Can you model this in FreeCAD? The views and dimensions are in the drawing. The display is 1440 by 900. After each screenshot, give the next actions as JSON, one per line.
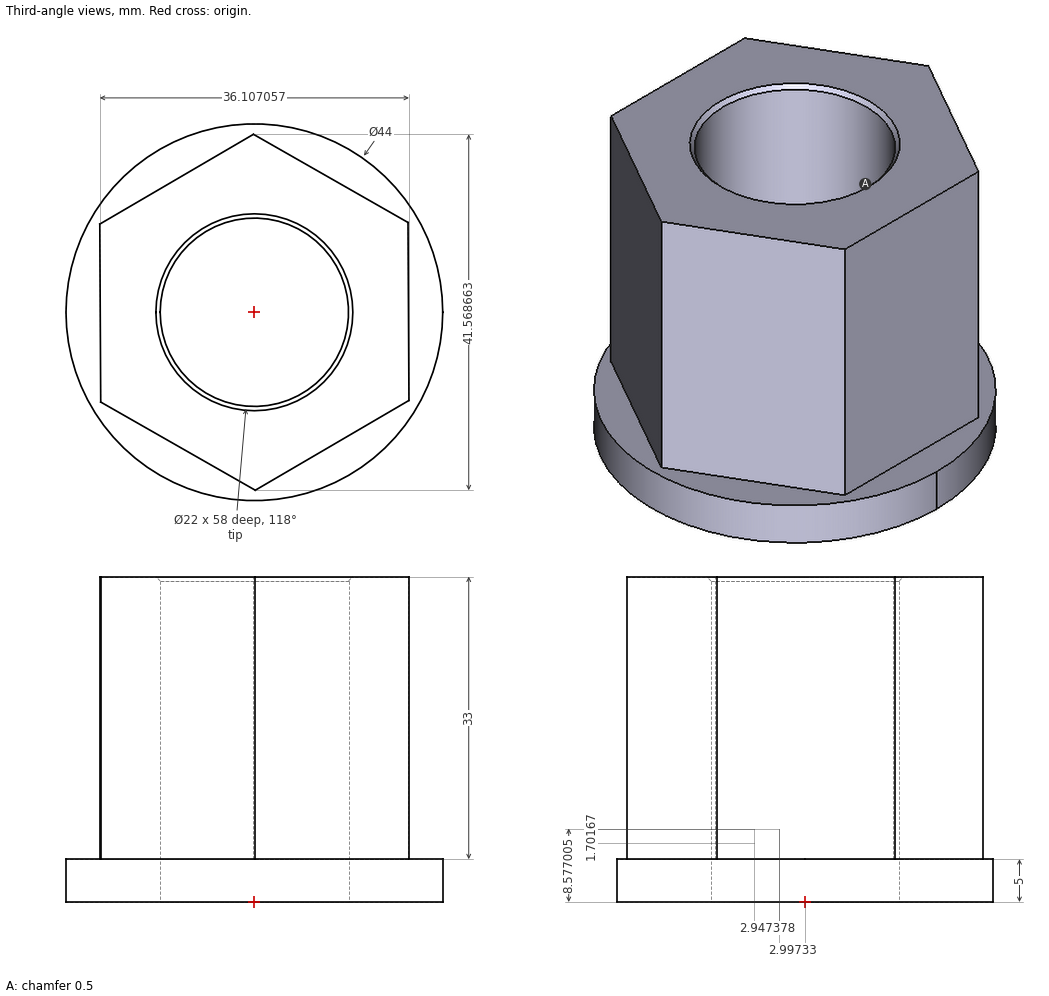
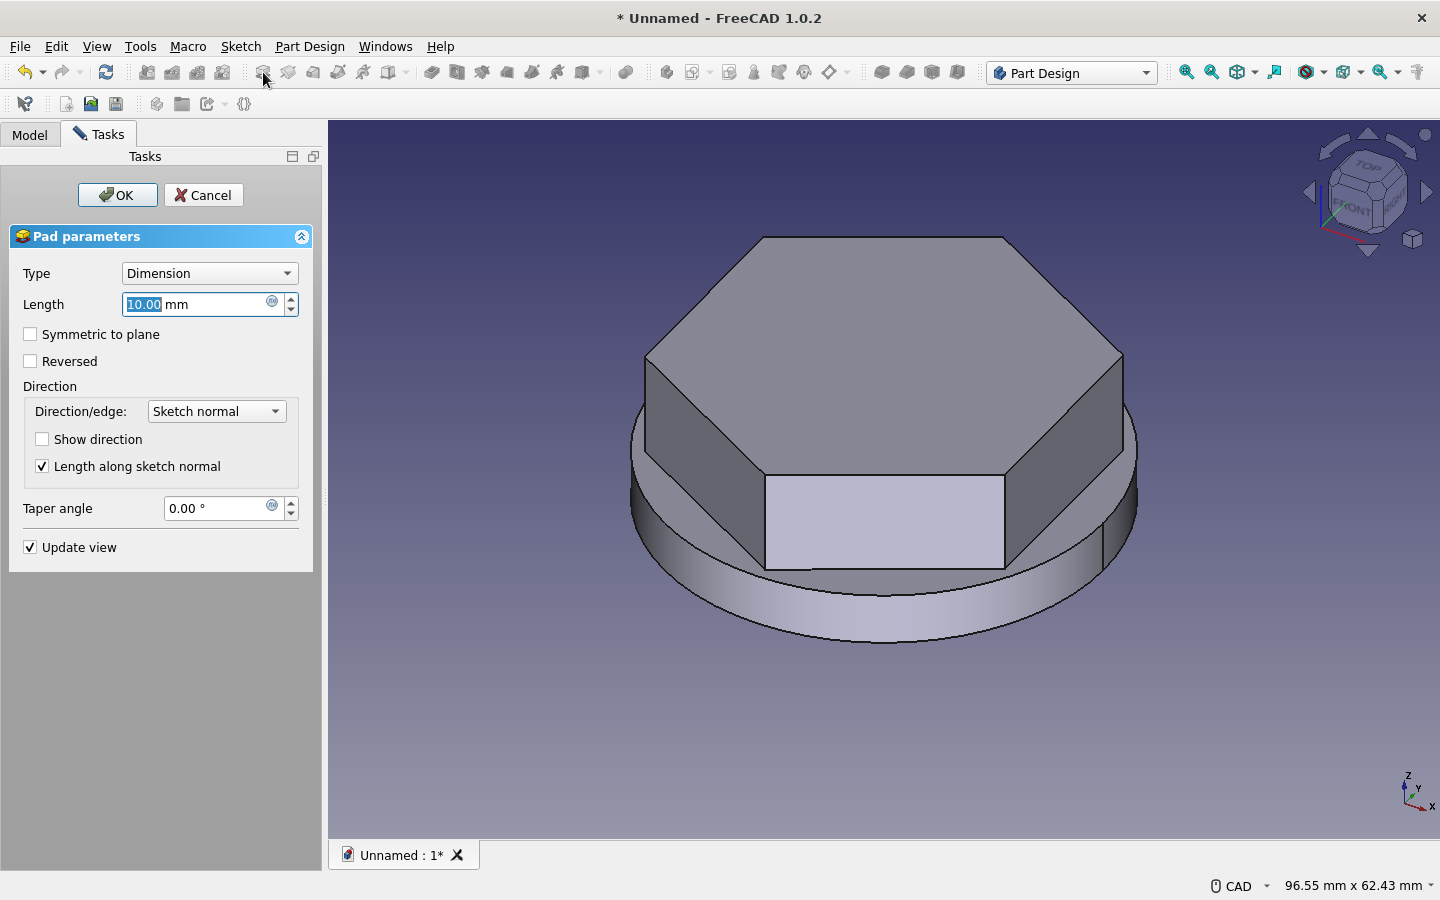
{"action": "type", "text": "33"}
{"action": "key", "text": "Tab"}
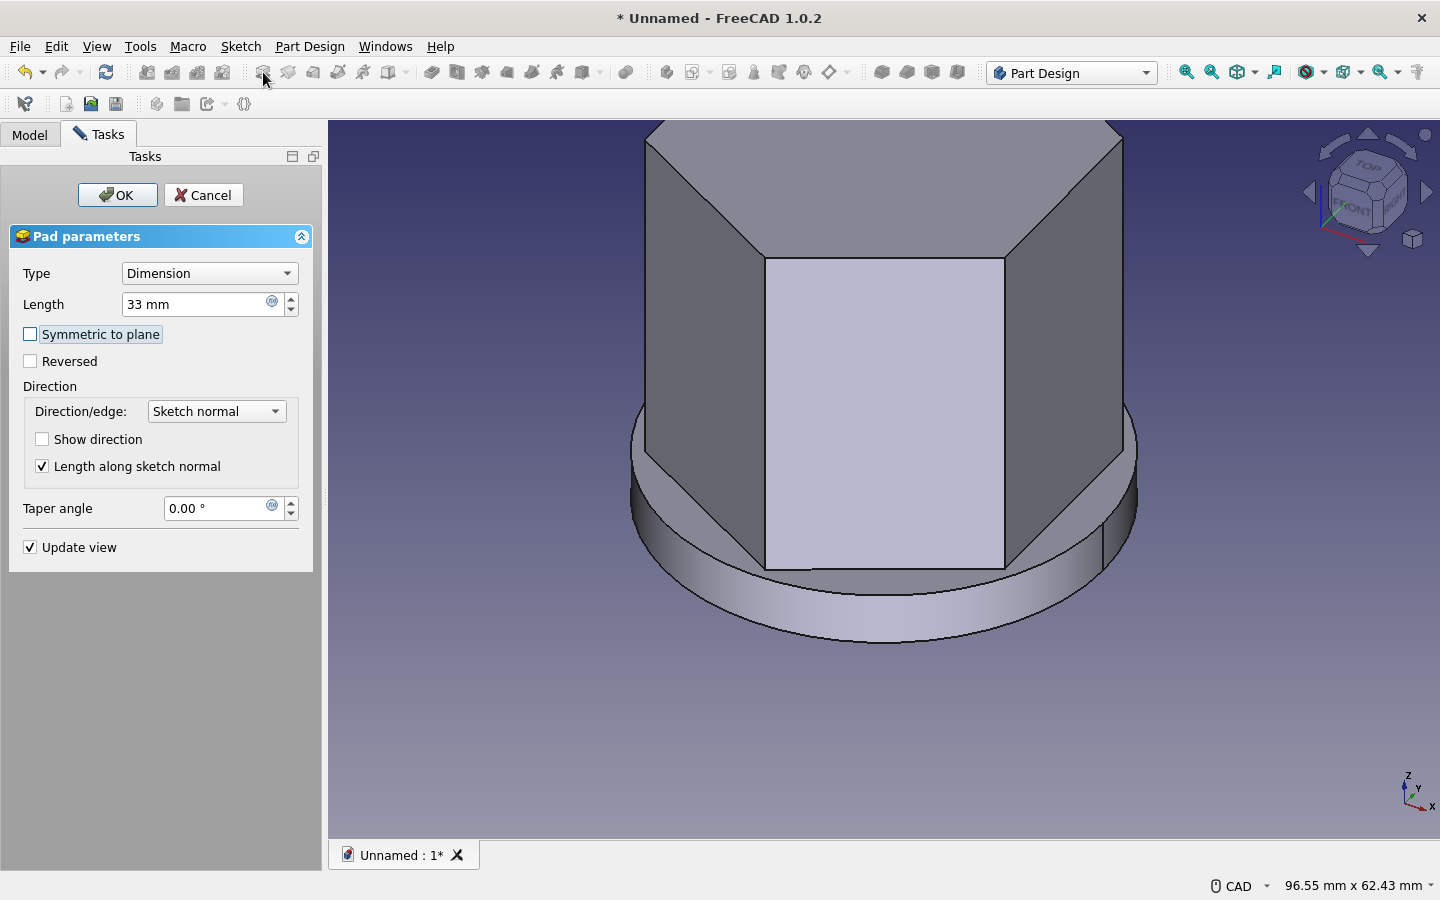
{"action": "left_click", "coordinate": [118, 195]}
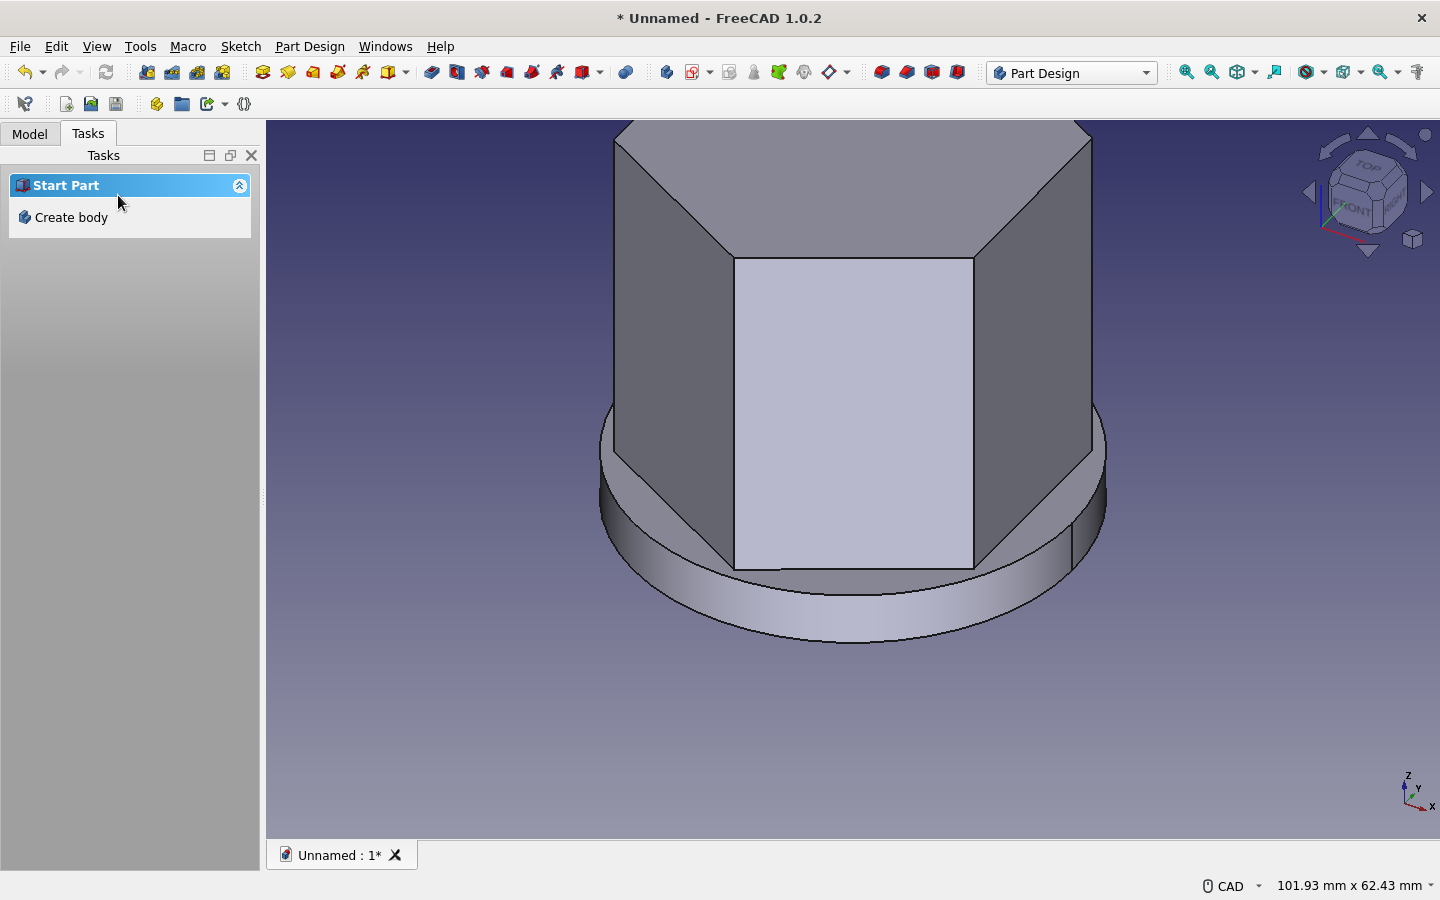
{"action": "key", "text": "v f"}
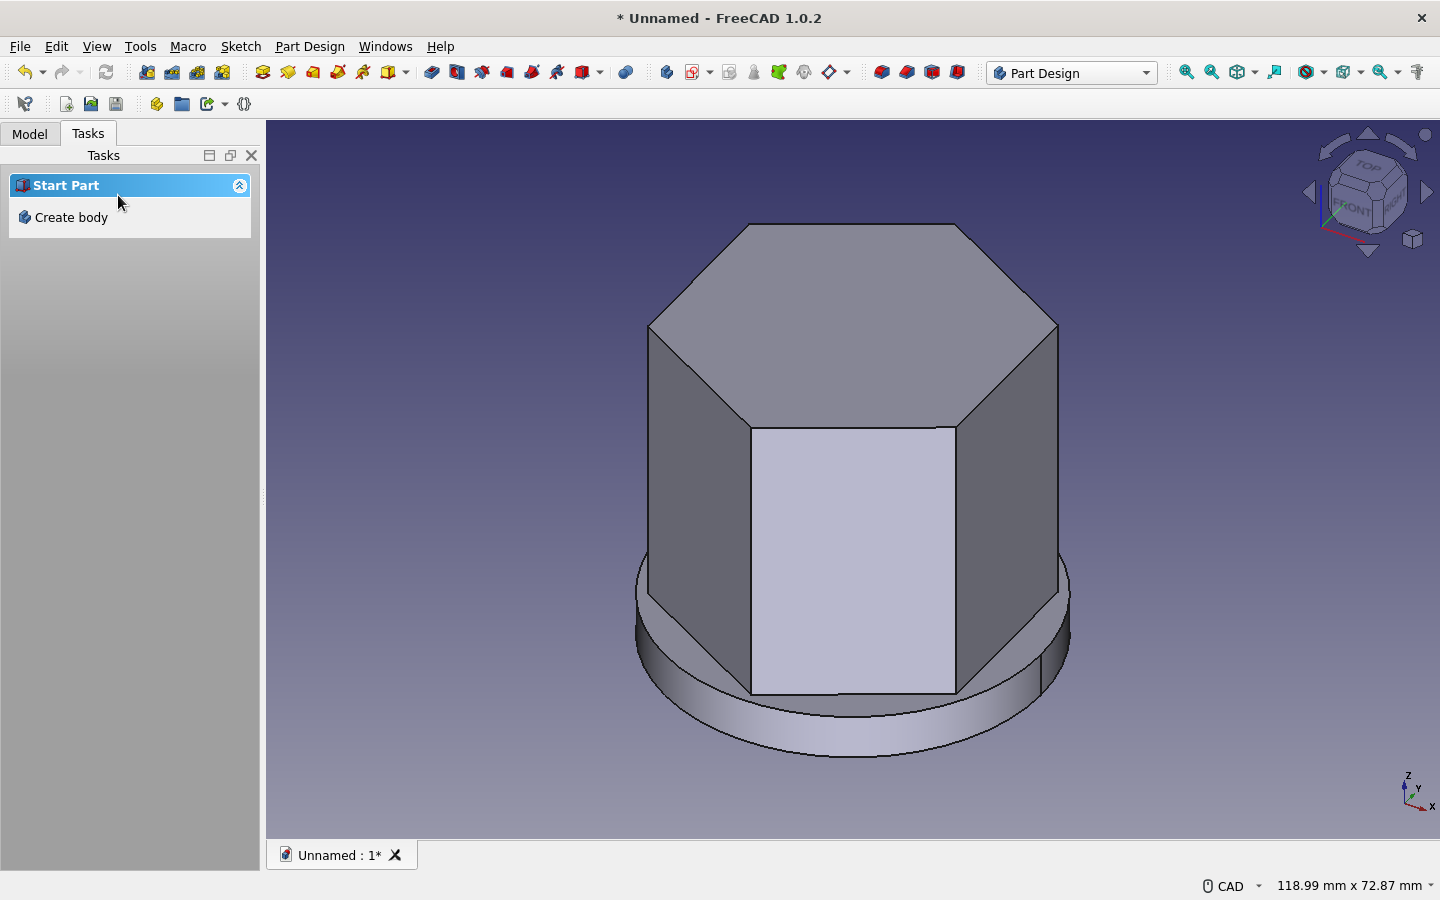
{"action": "left_click", "coordinate": [692, 72]}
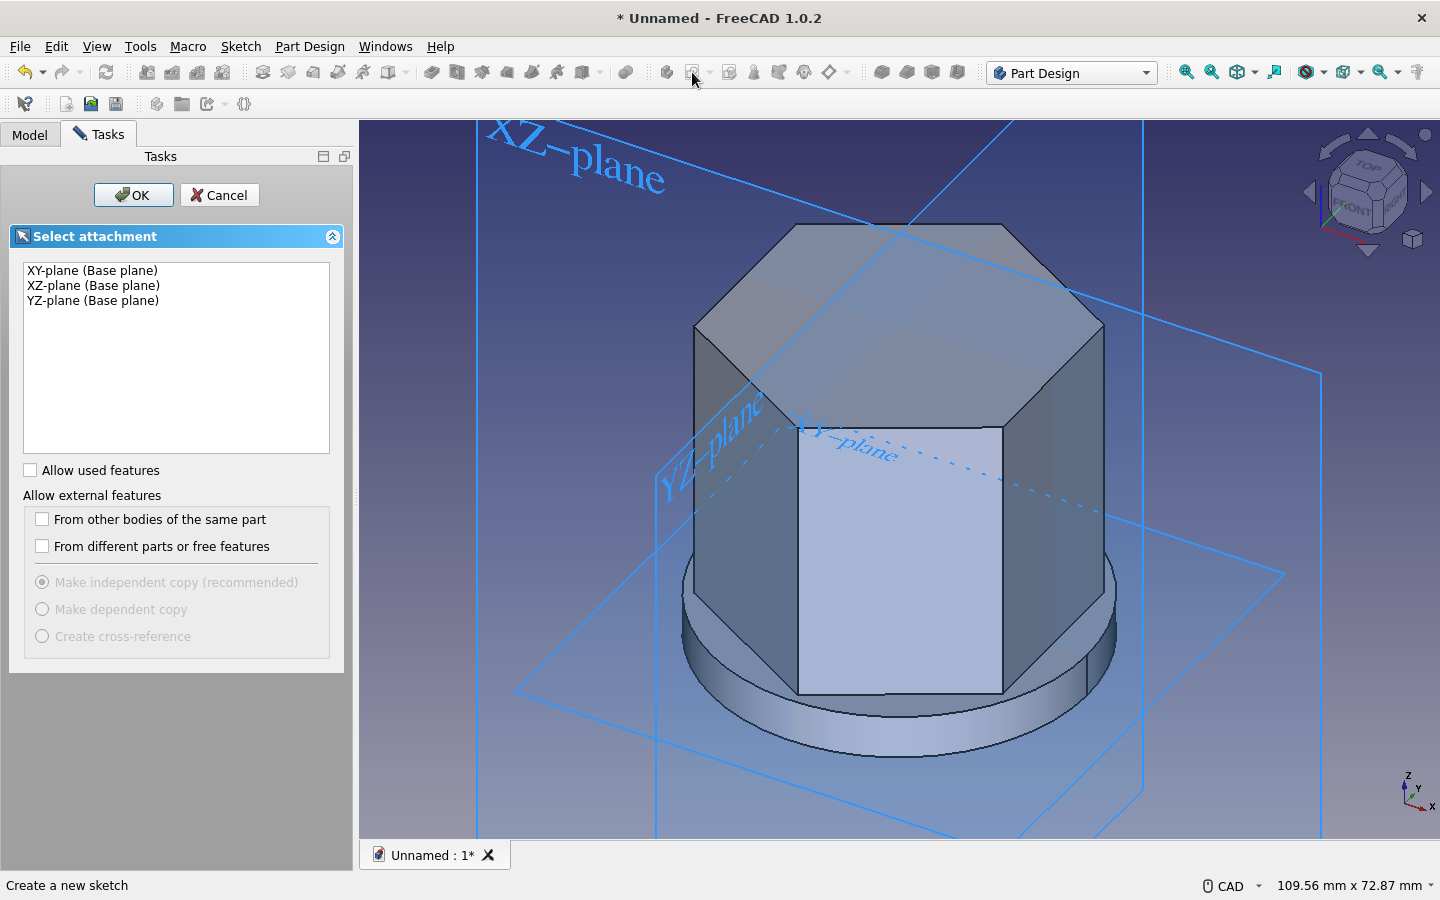
{"action": "left_click", "coordinate": [84, 300]}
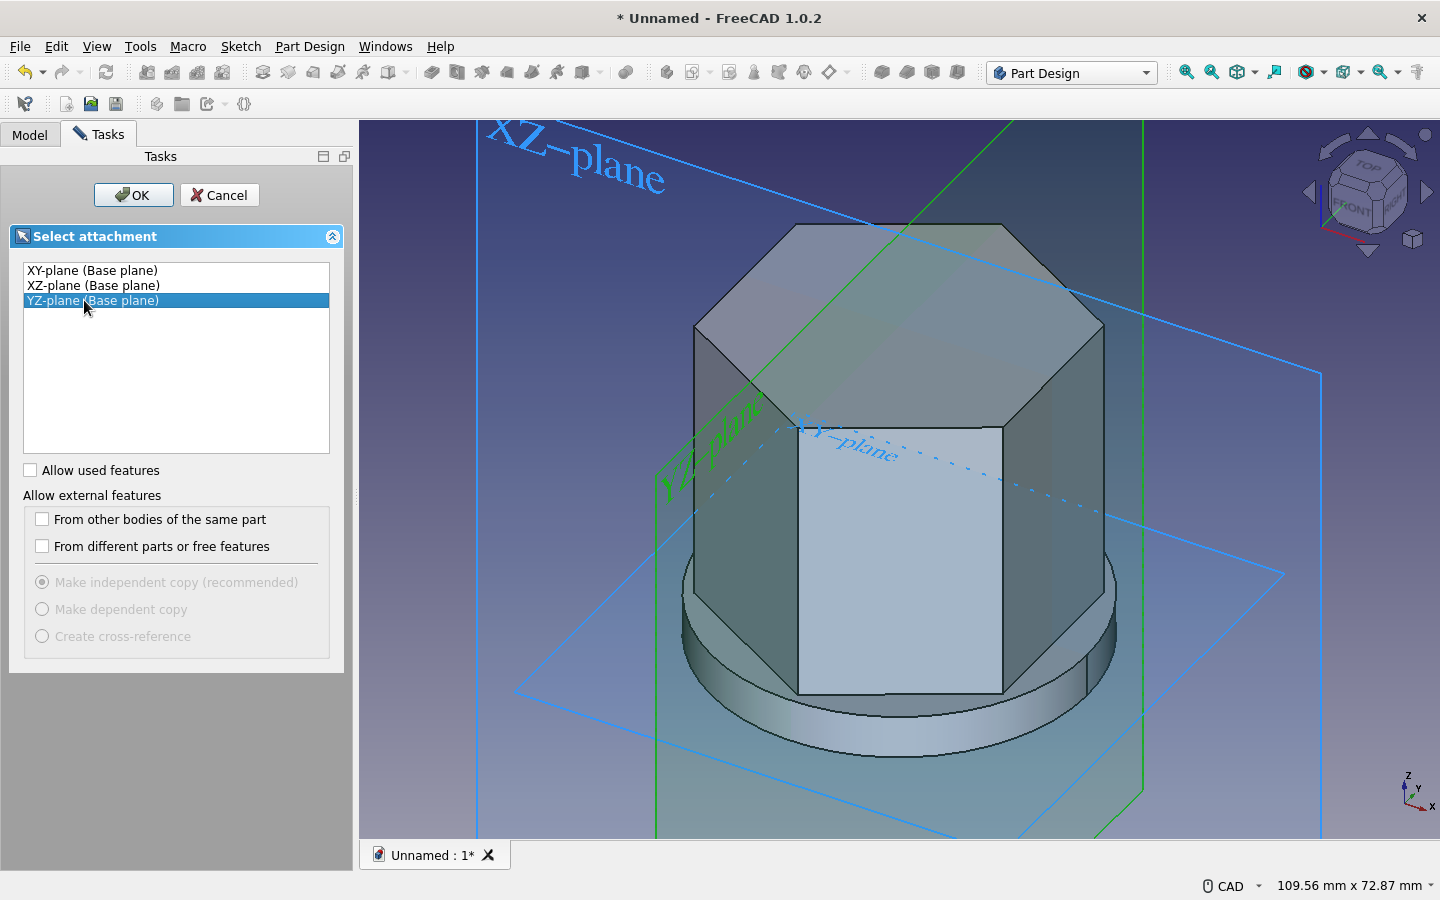
{"action": "left_click", "coordinate": [134, 195]}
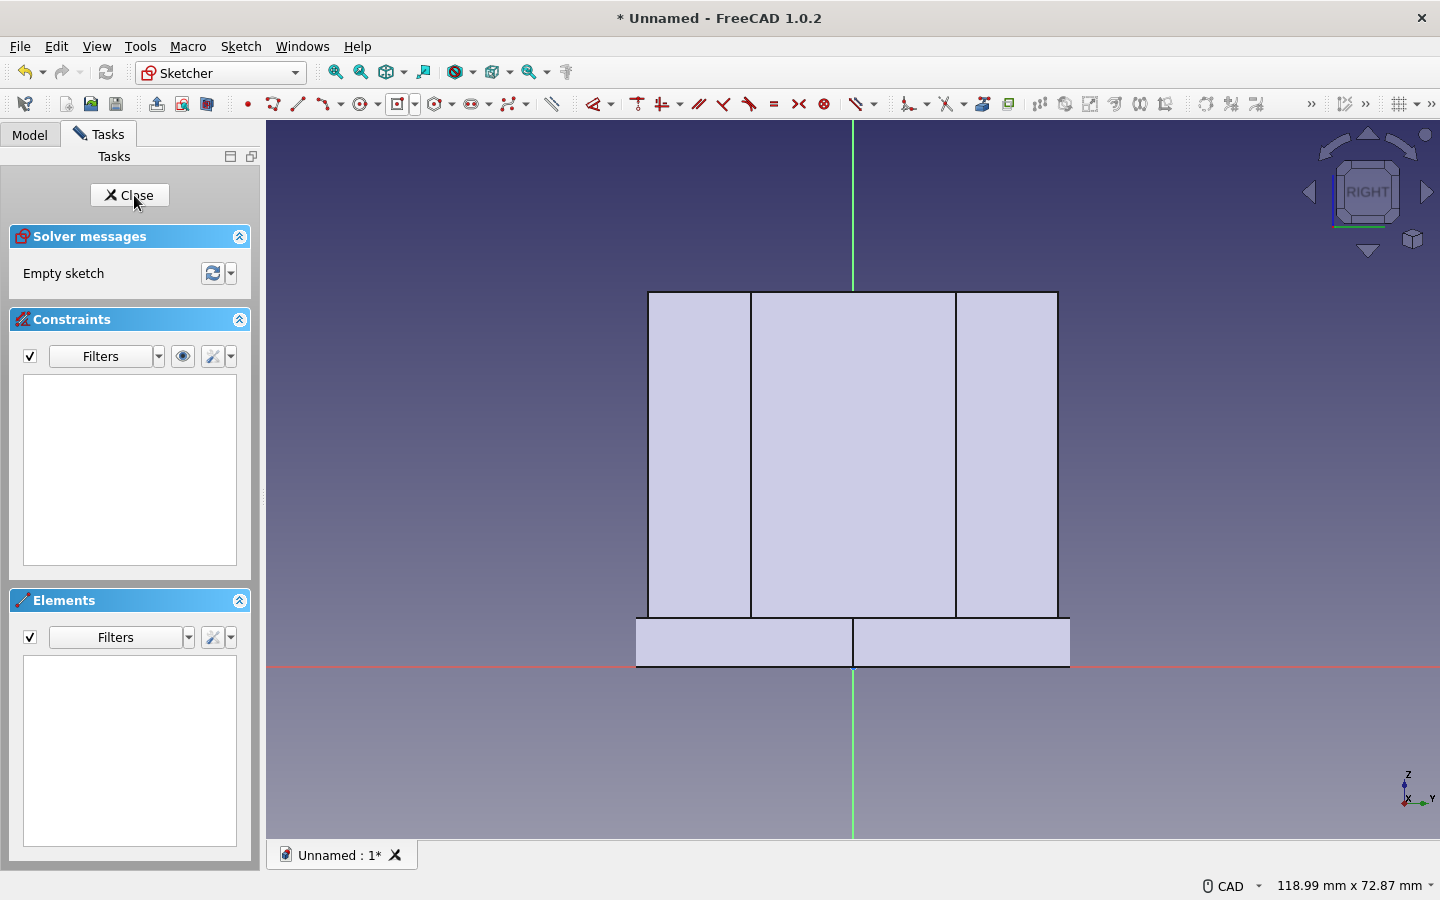
{"action": "key", "text": "q s"}